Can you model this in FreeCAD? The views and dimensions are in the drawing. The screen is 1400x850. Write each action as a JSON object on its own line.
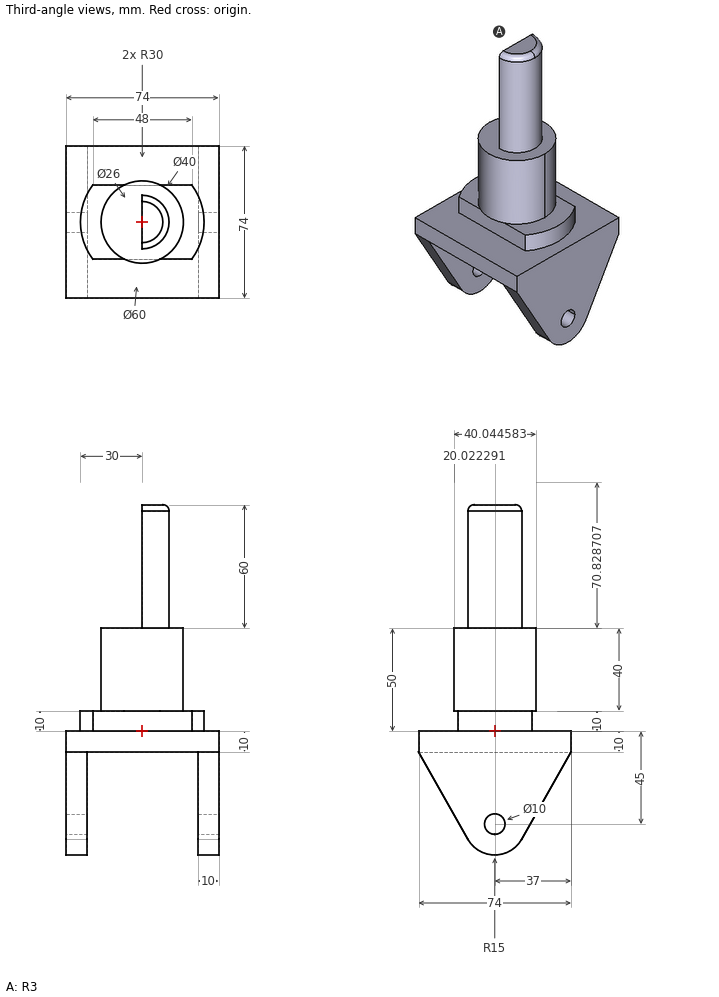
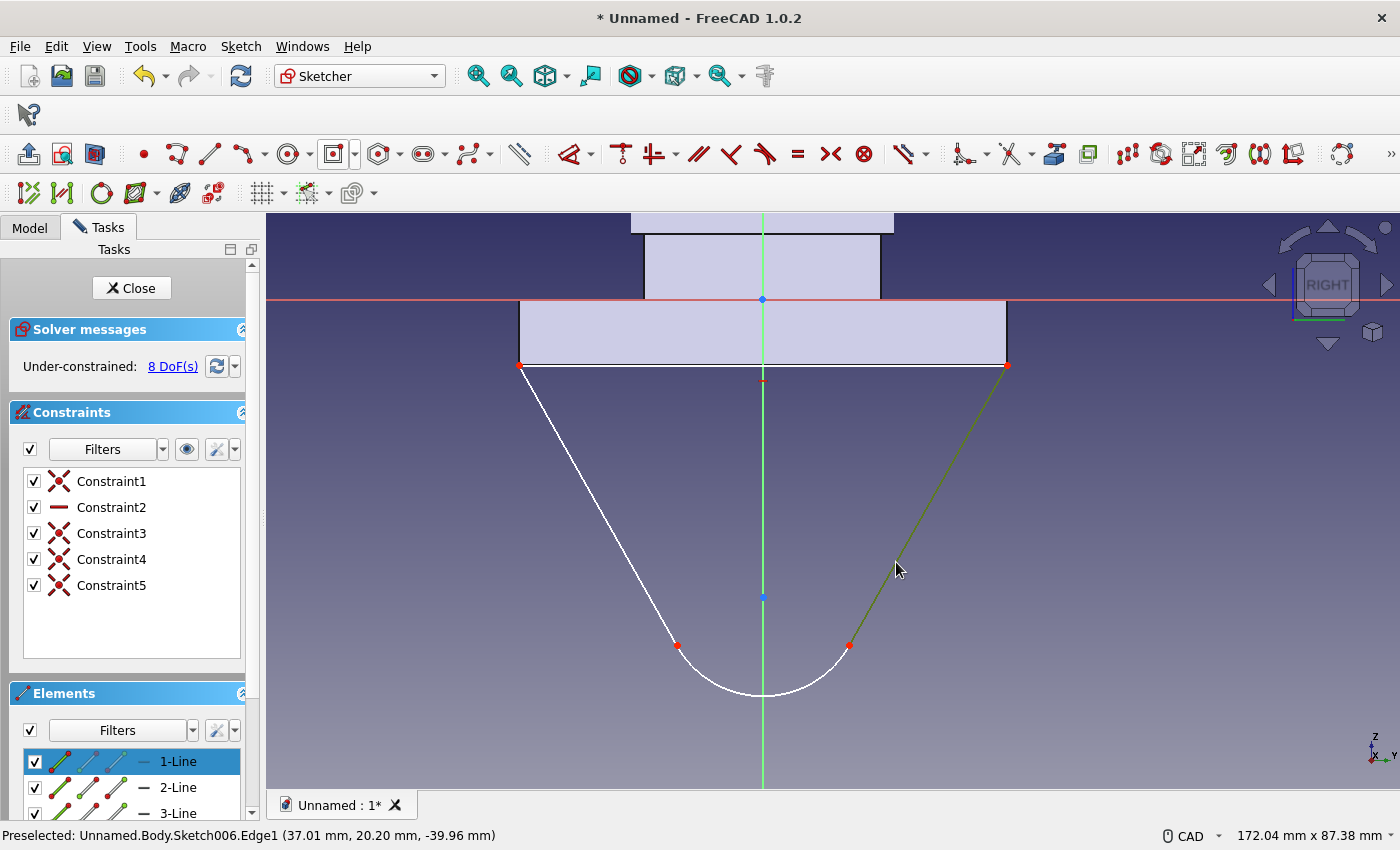
{"action": "left_click", "coordinate": [722, 688]}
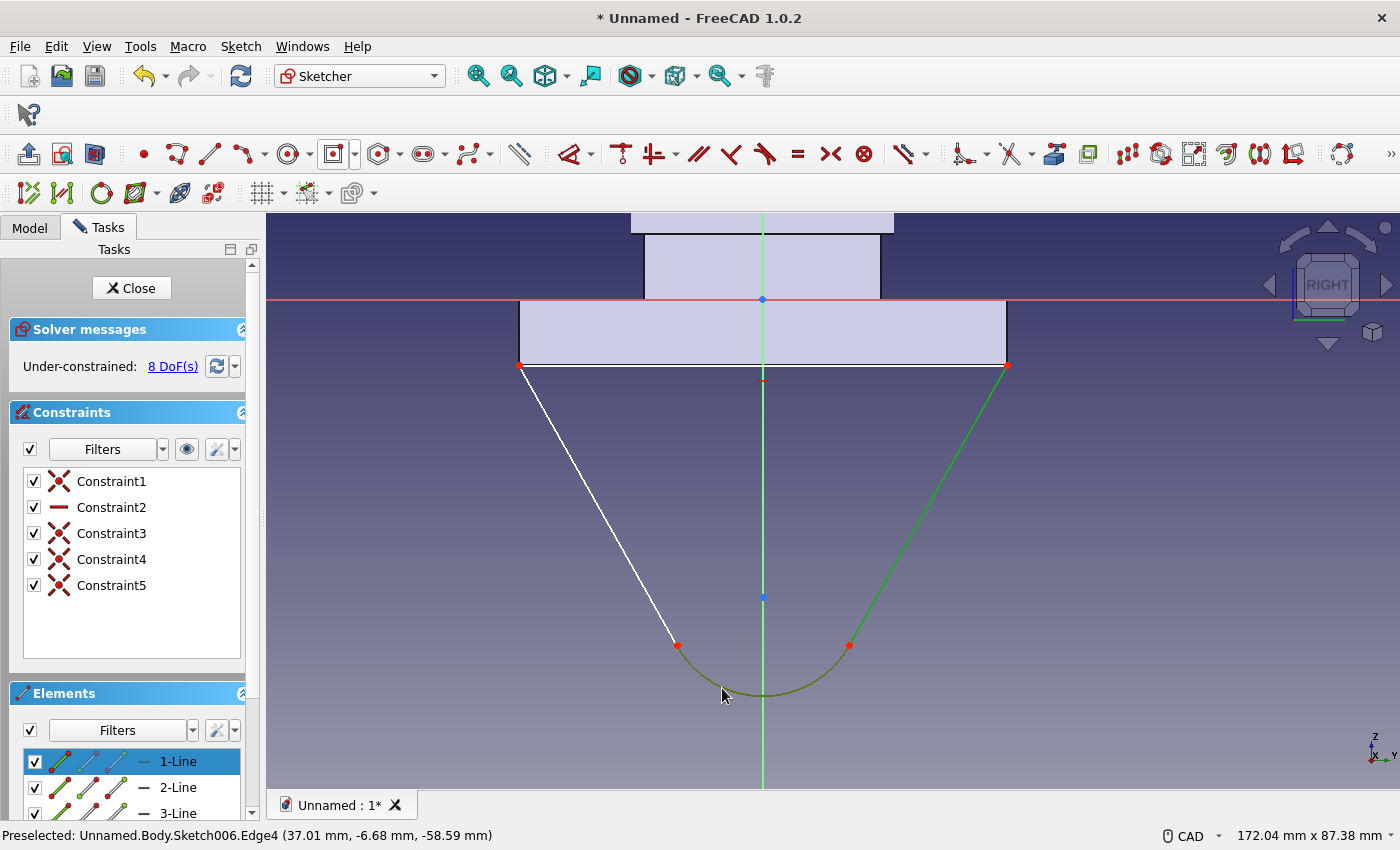
{"action": "key", "text": "t"}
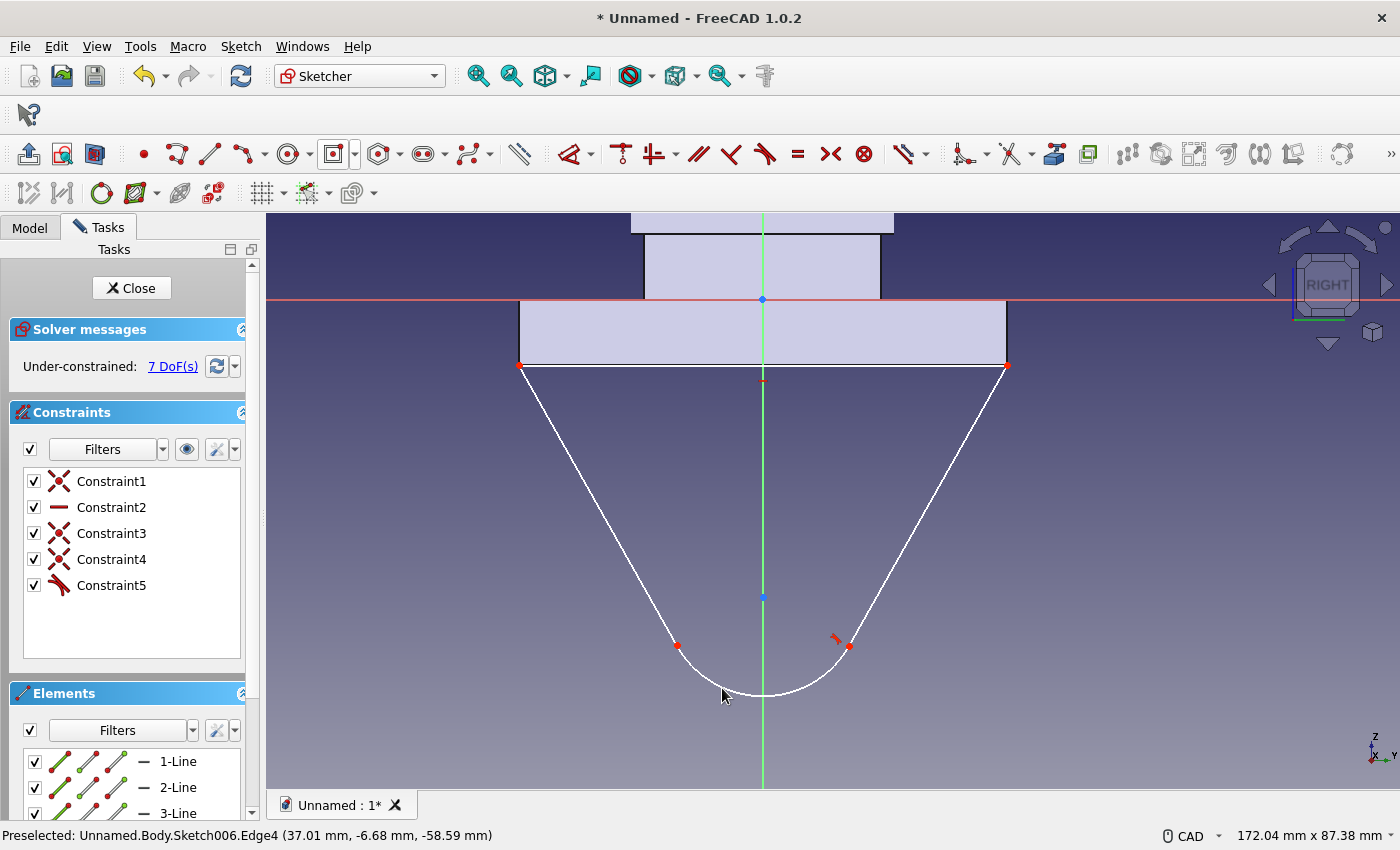
{"action": "left_click", "coordinate": [566, 450]}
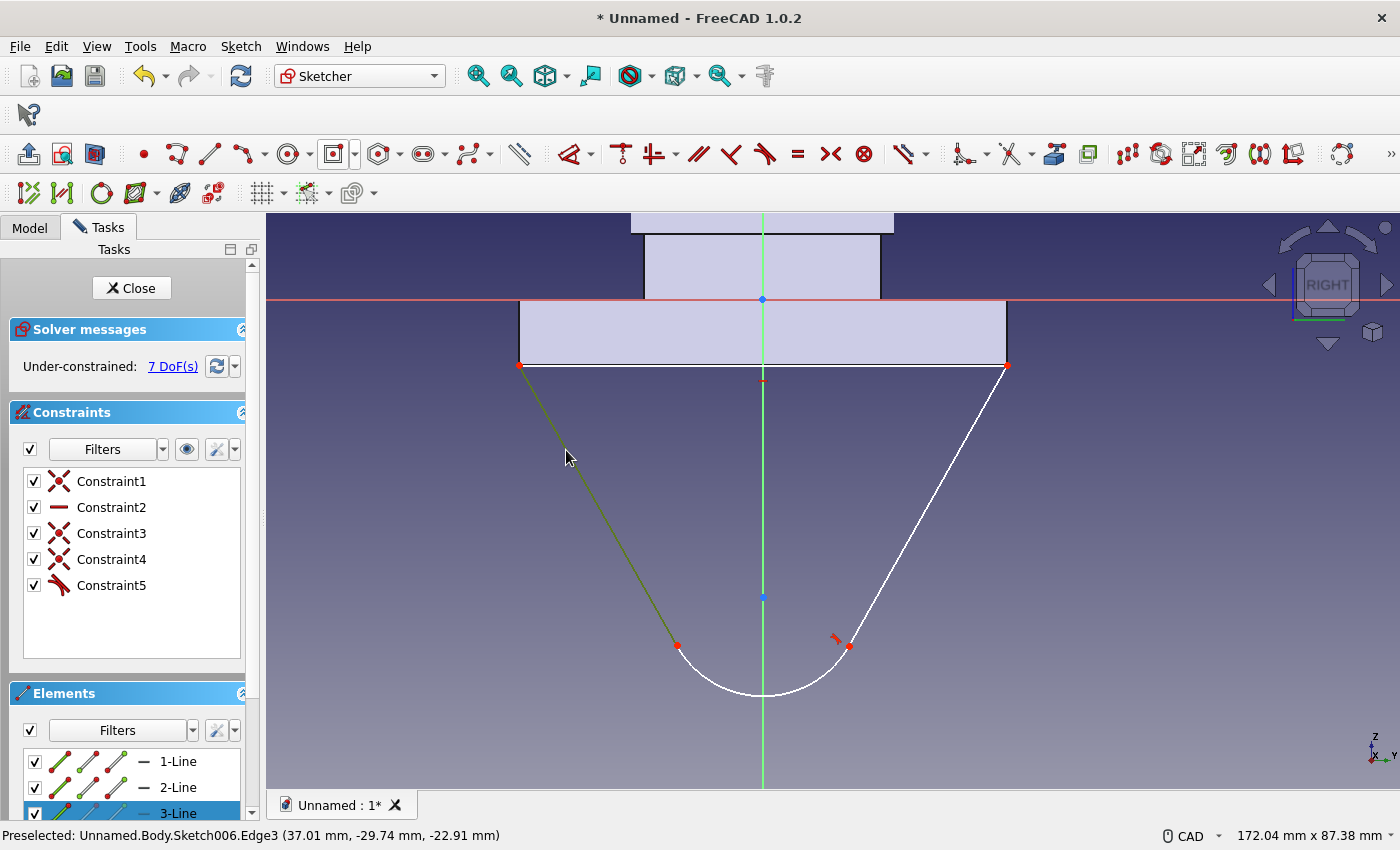
{"action": "left_click", "coordinate": [722, 688]}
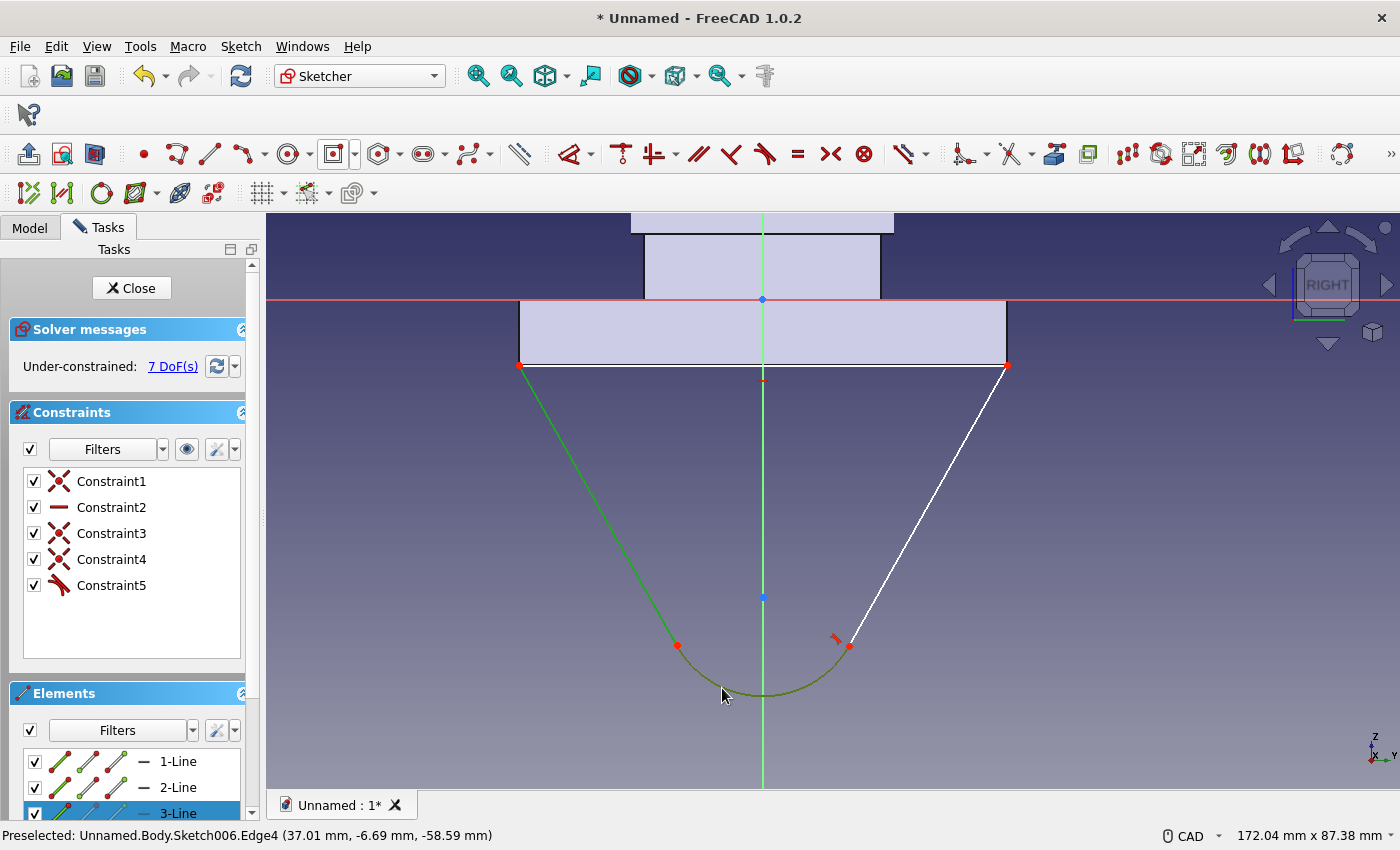
{"action": "left_click", "coordinate": [765, 154]}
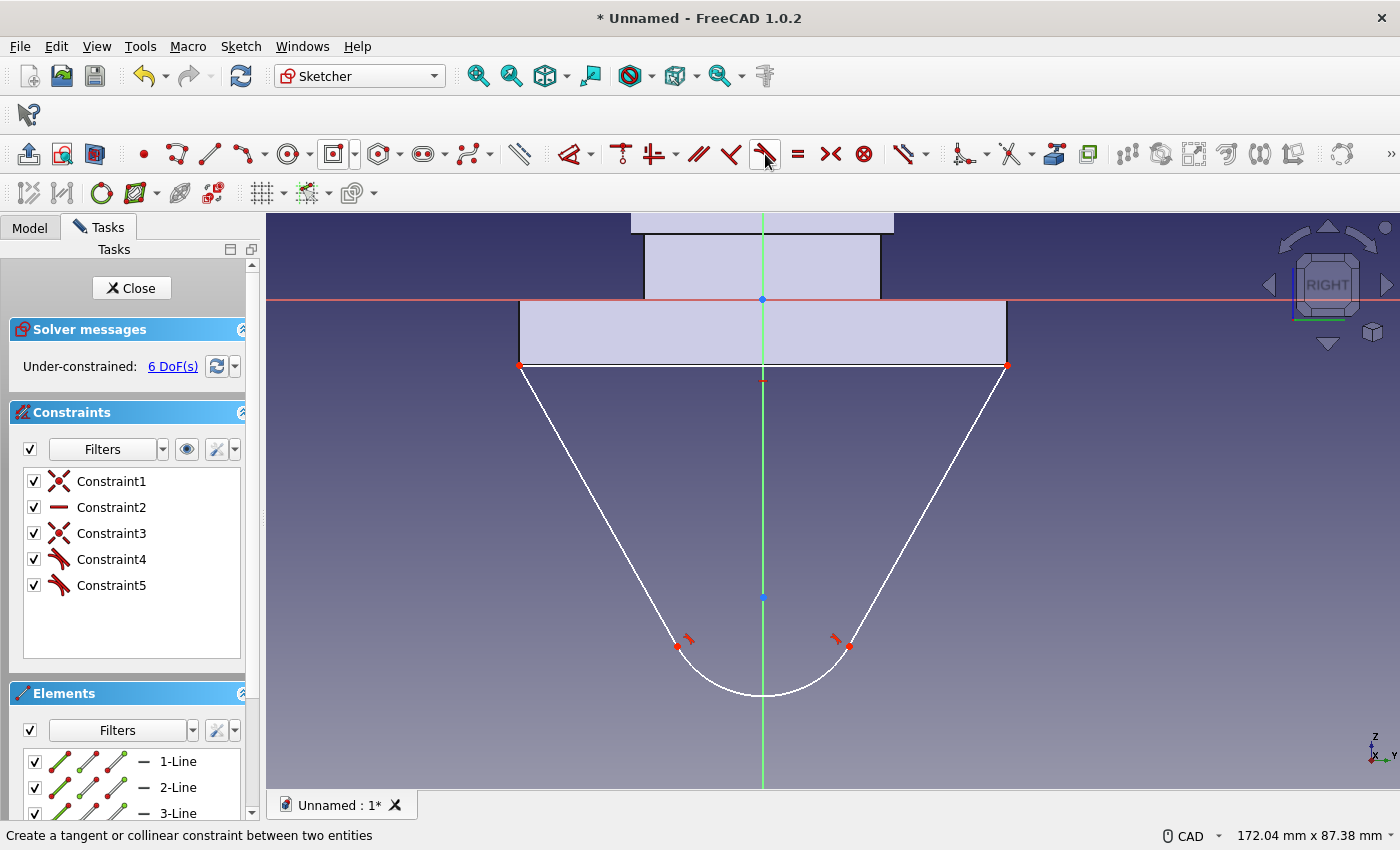
{"action": "left_click", "coordinate": [763, 598]}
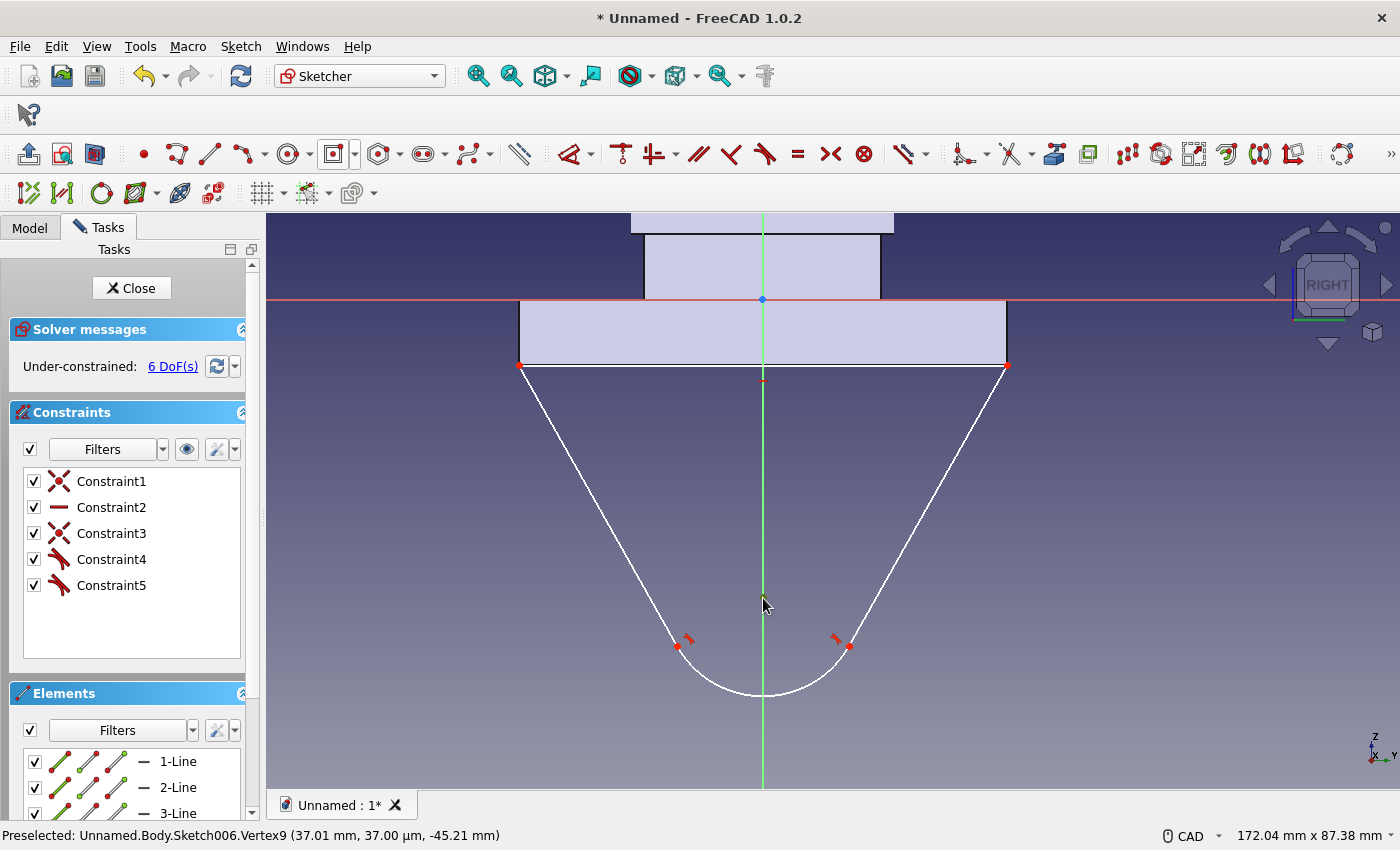
{"action": "left_click", "coordinate": [763, 650]}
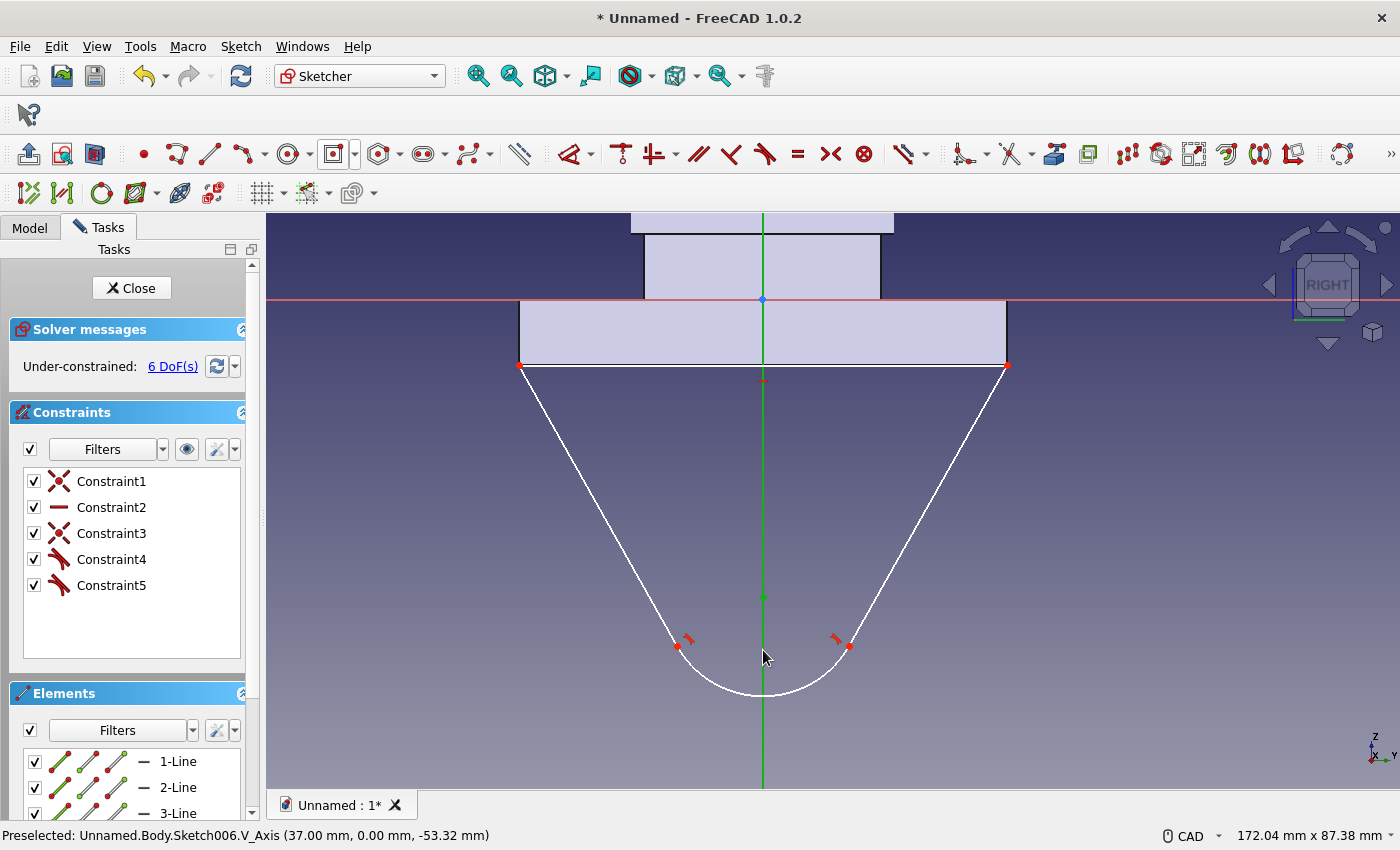
{"action": "key", "text": "c"}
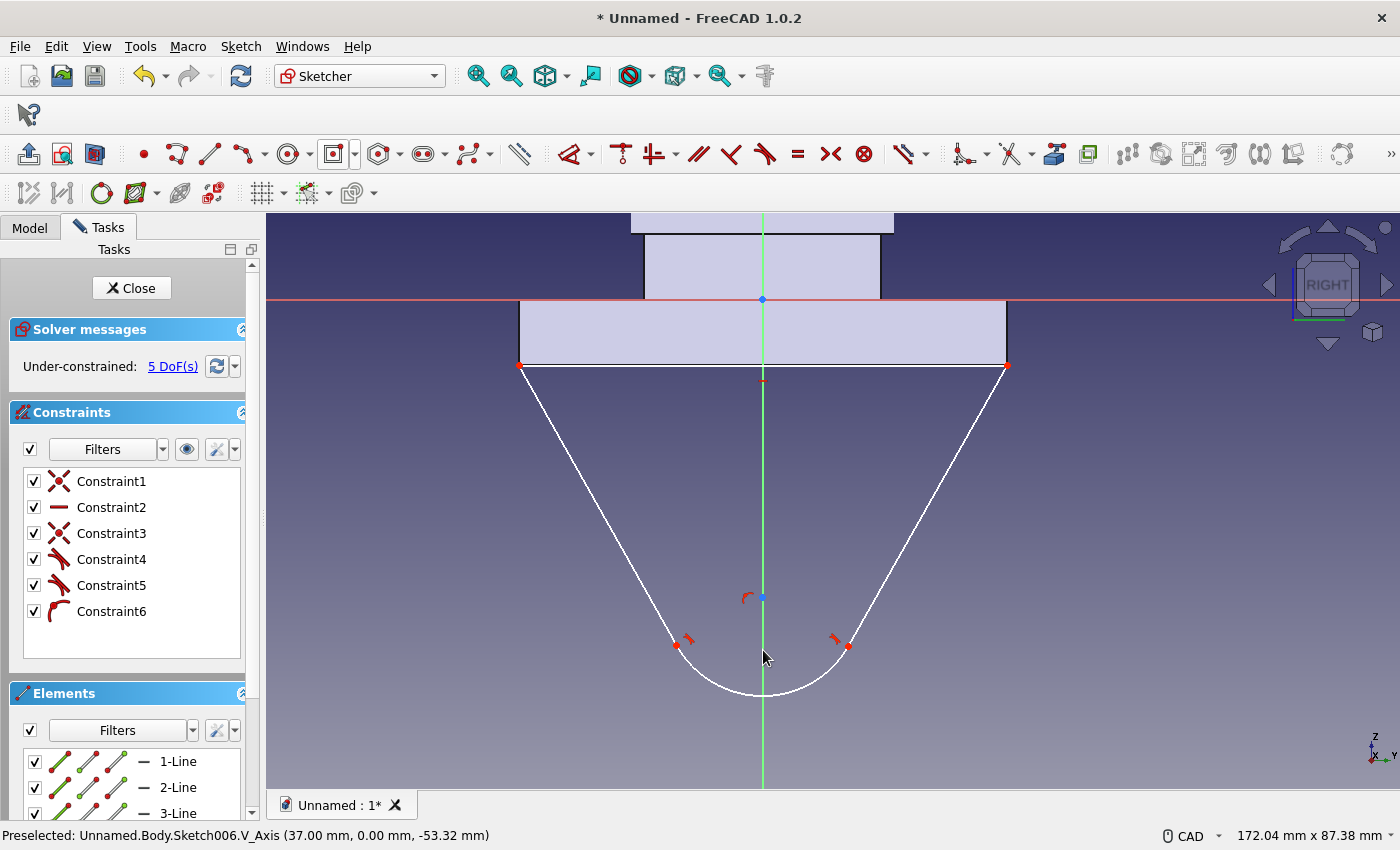
{"action": "key", "text": "d"}